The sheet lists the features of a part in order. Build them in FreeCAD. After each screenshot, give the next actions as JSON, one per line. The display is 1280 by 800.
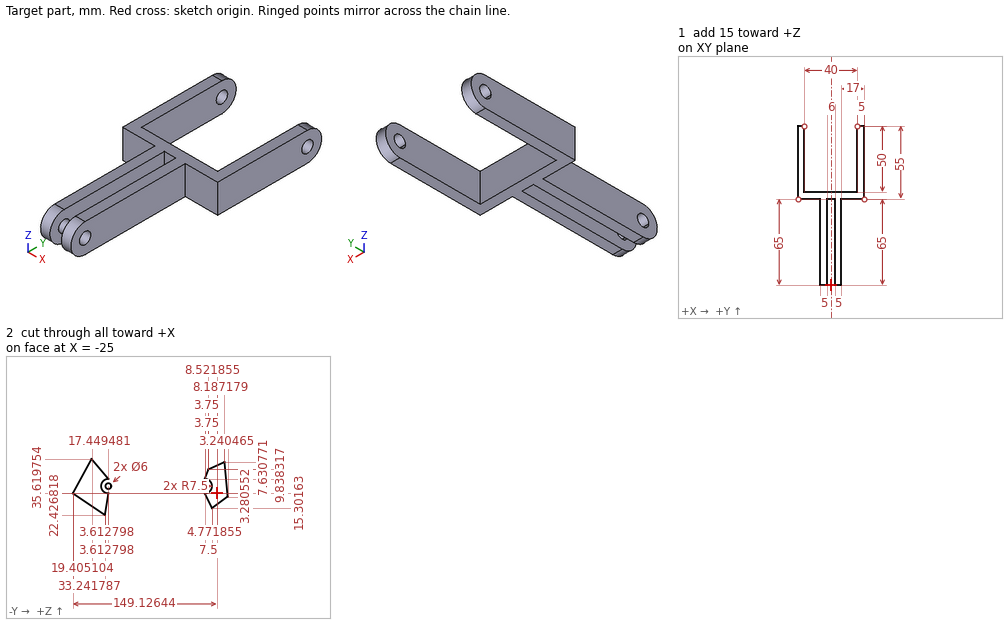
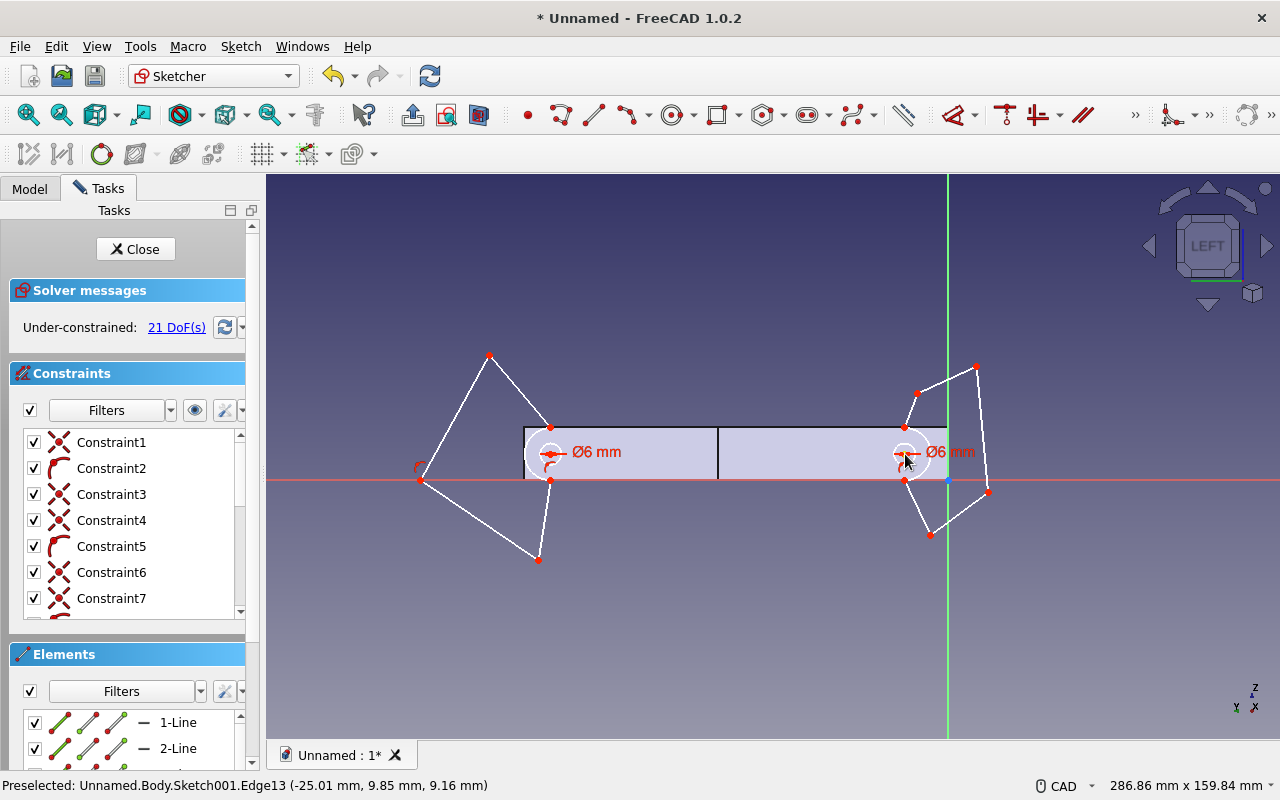
{"action": "left_click", "coordinate": [530, 439]}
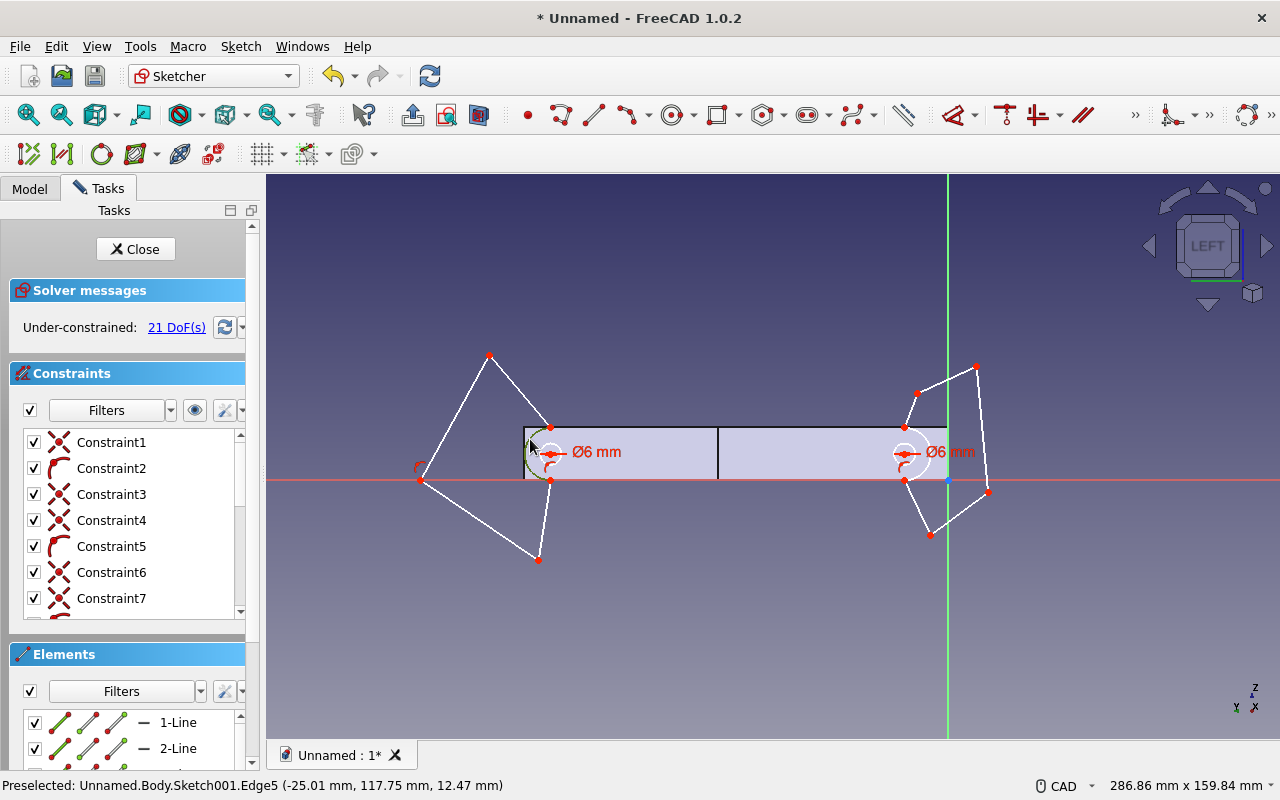
{"action": "scroll", "coordinate": [926, 469], "scroll_direction": "up", "scroll_amount": 2}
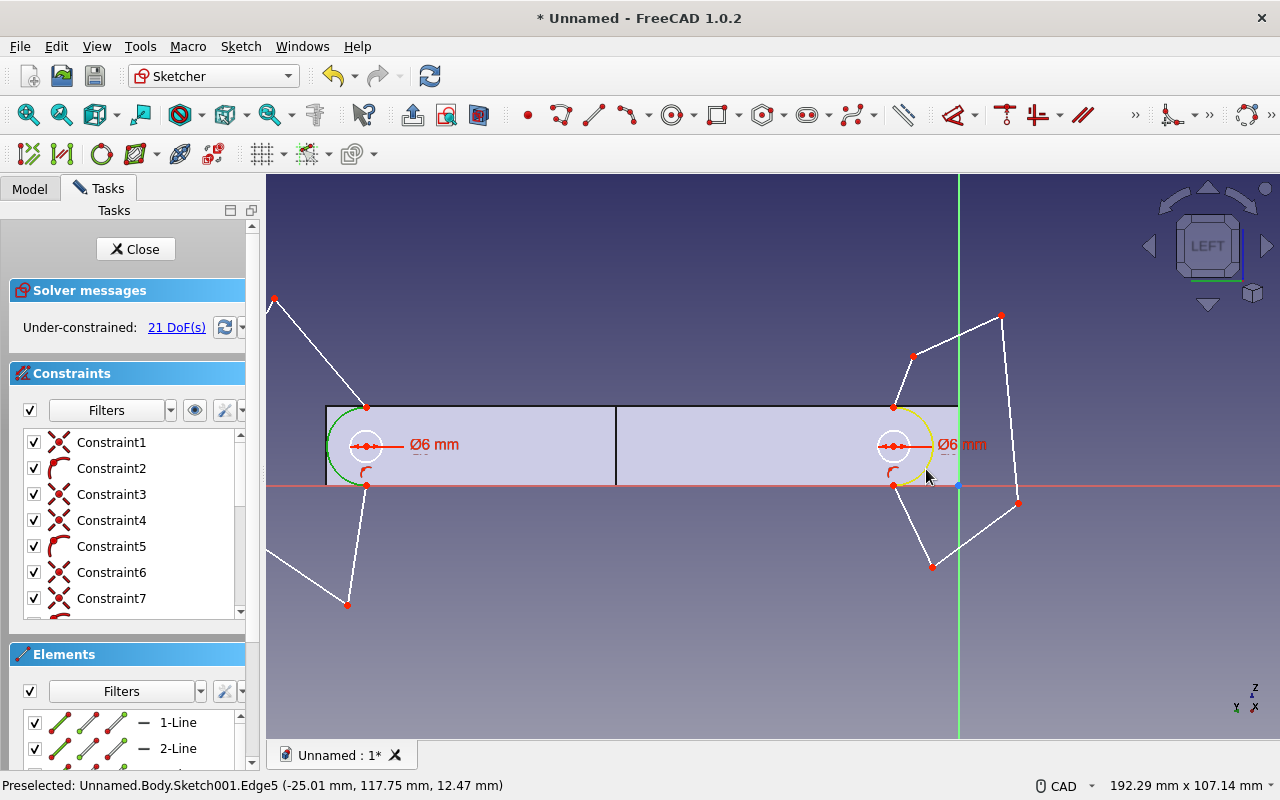
{"action": "left_click", "coordinate": [925, 469]}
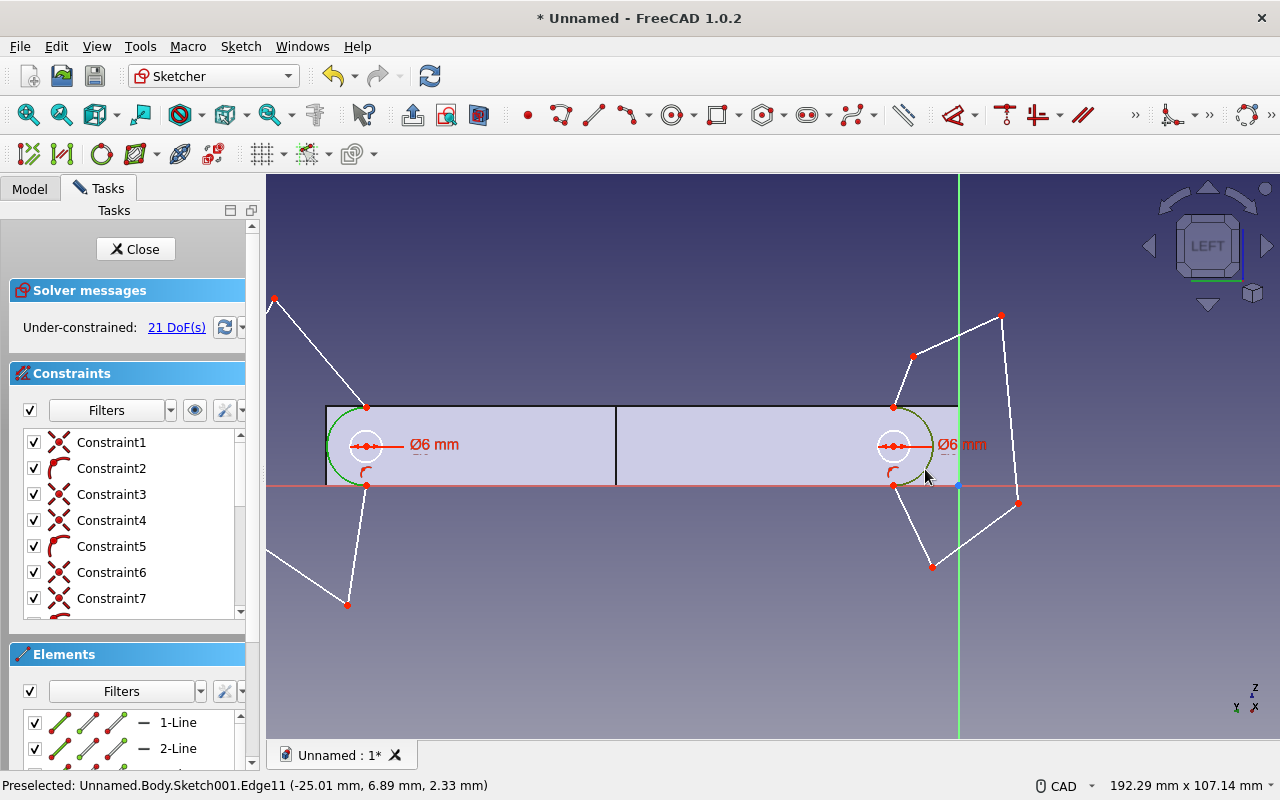
{"action": "key", "text": "e"}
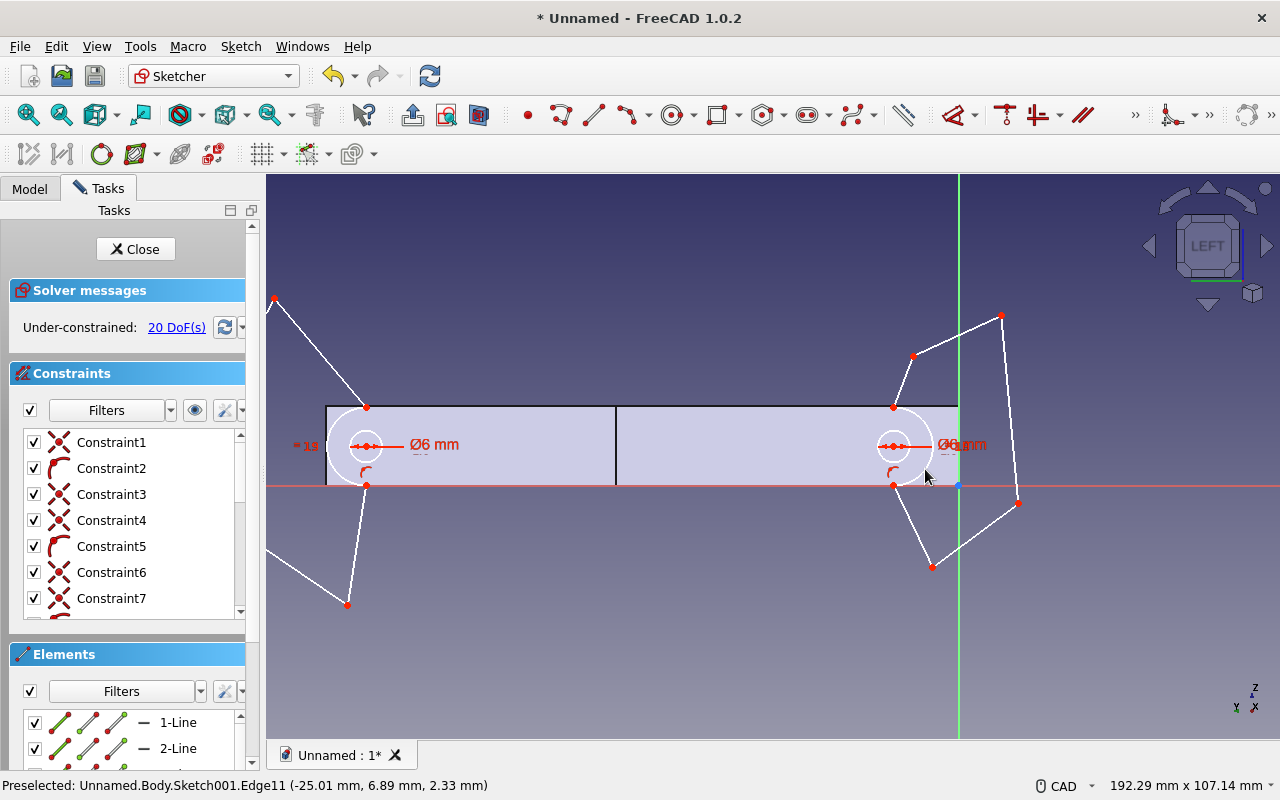
{"action": "key", "text": "d"}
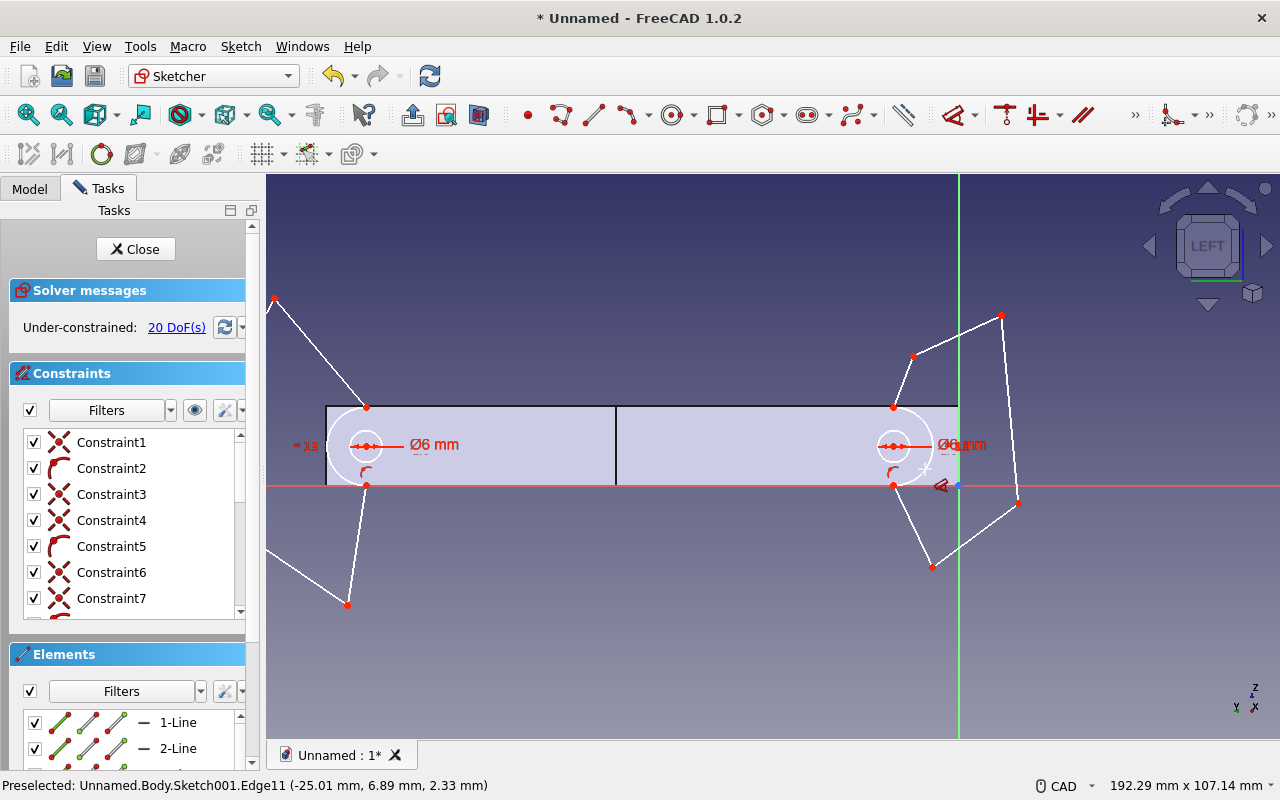
{"action": "left_click", "coordinate": [334, 424]}
{"action": "left_click", "coordinate": [308, 406]}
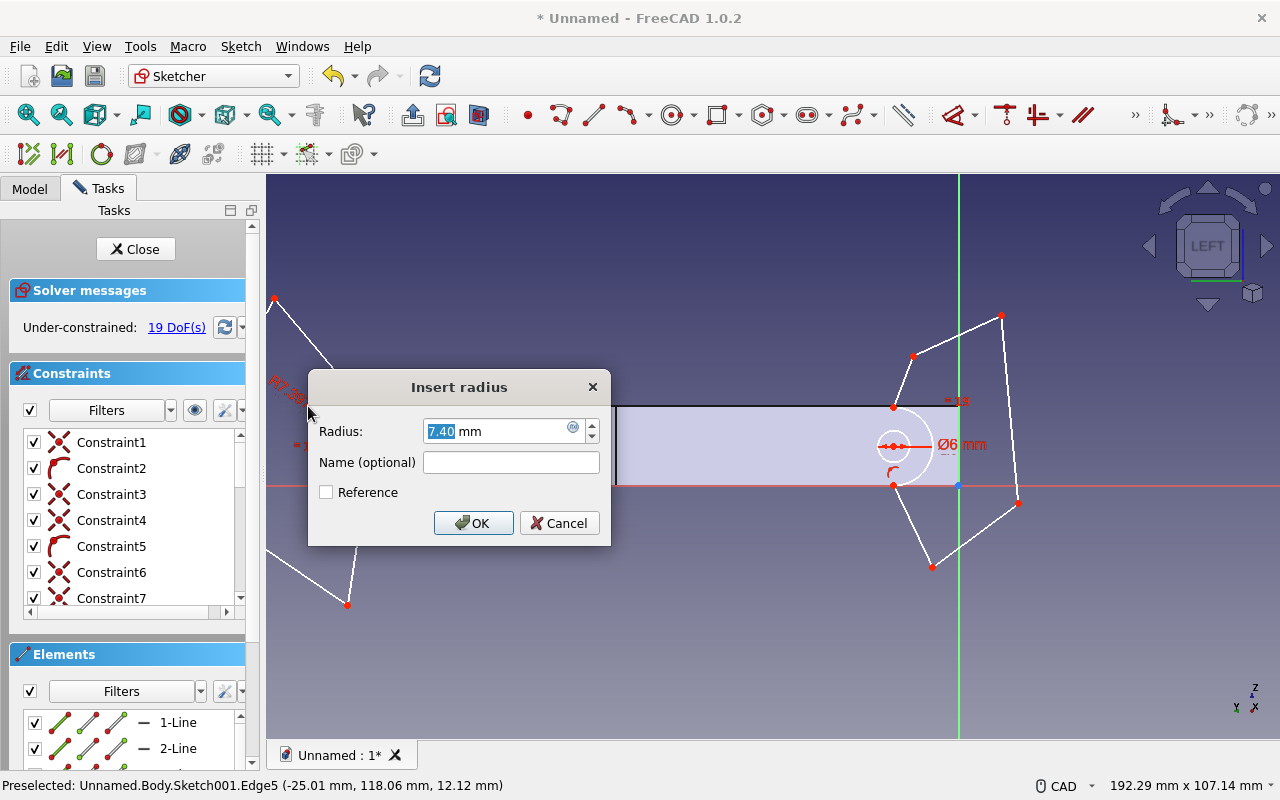
{"action": "type", "text": "7.5"}
{"action": "key", "text": "Return"}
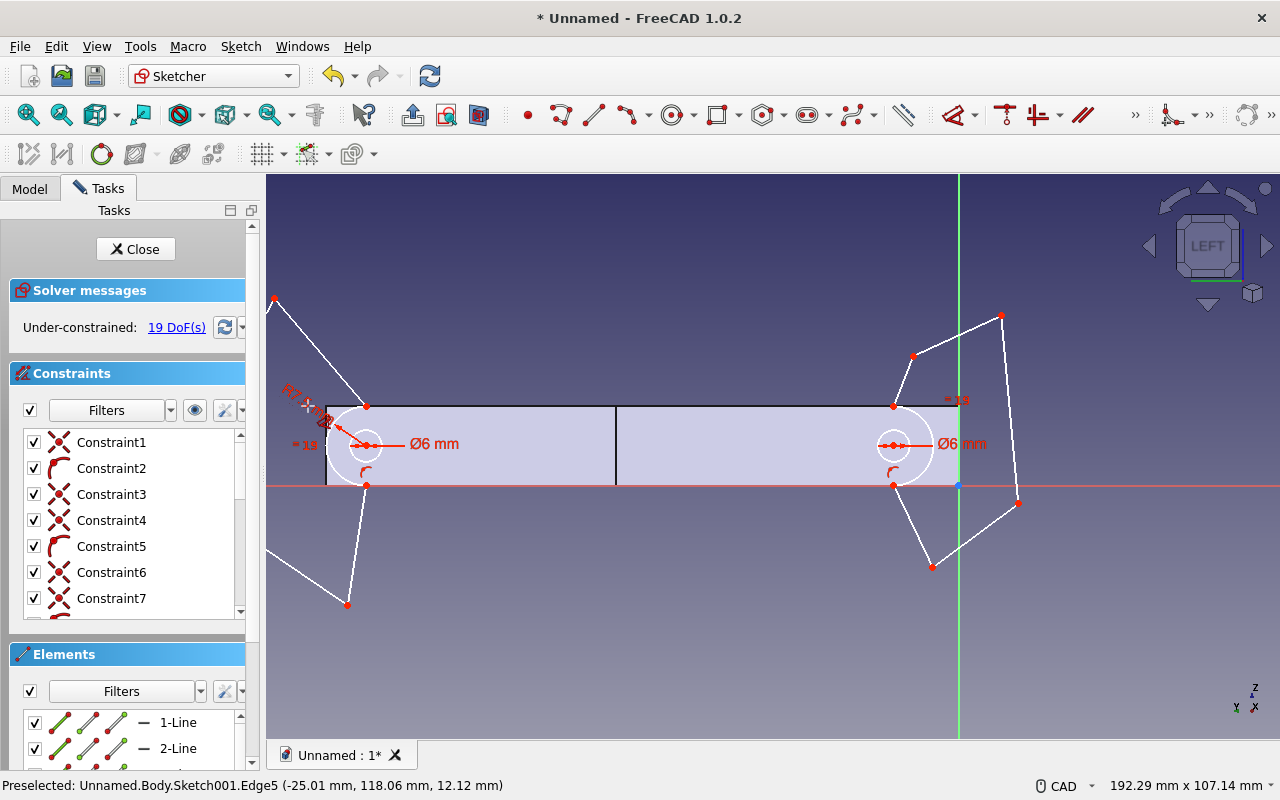
{"action": "left_click", "coordinate": [905, 510]}
{"action": "left_click", "coordinate": [913, 602]}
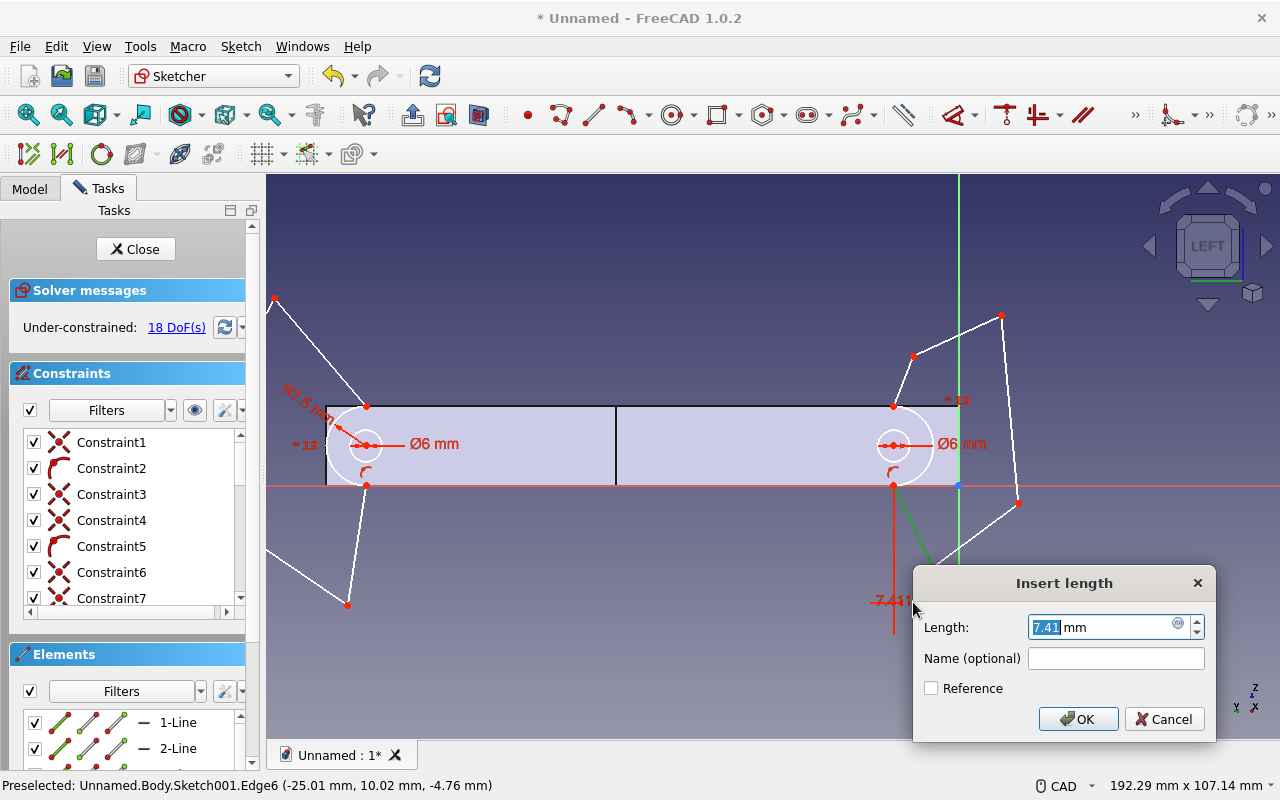
{"action": "type", "text": "7.5"}
{"action": "key", "text": "Return"}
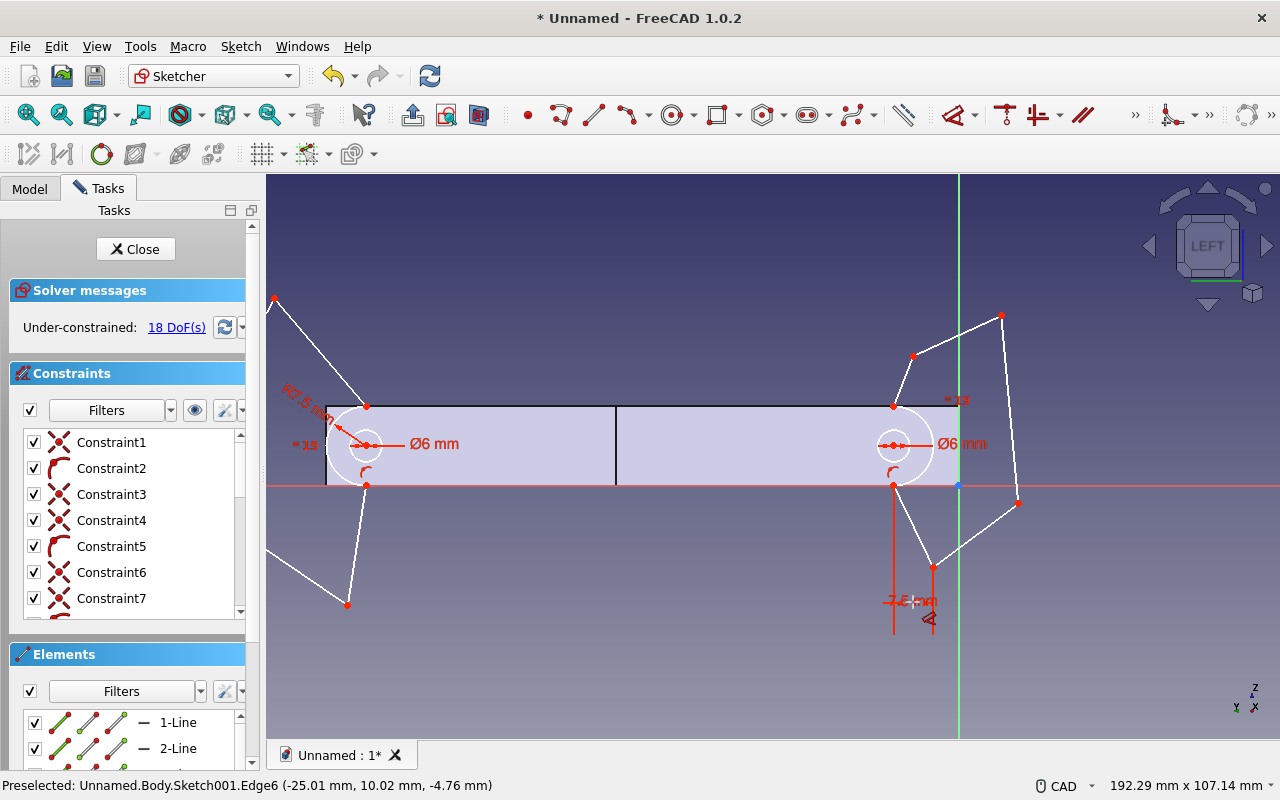
{"action": "scroll", "coordinate": [907, 371], "scroll_direction": "up", "scroll_amount": 4}